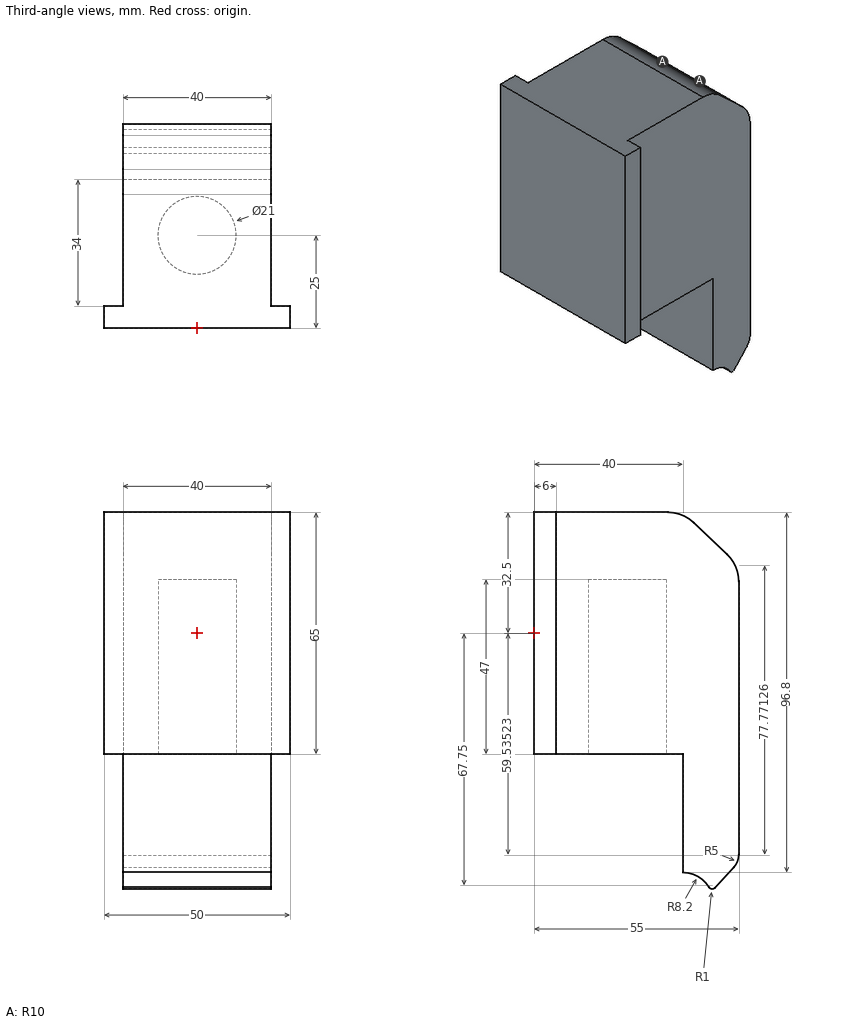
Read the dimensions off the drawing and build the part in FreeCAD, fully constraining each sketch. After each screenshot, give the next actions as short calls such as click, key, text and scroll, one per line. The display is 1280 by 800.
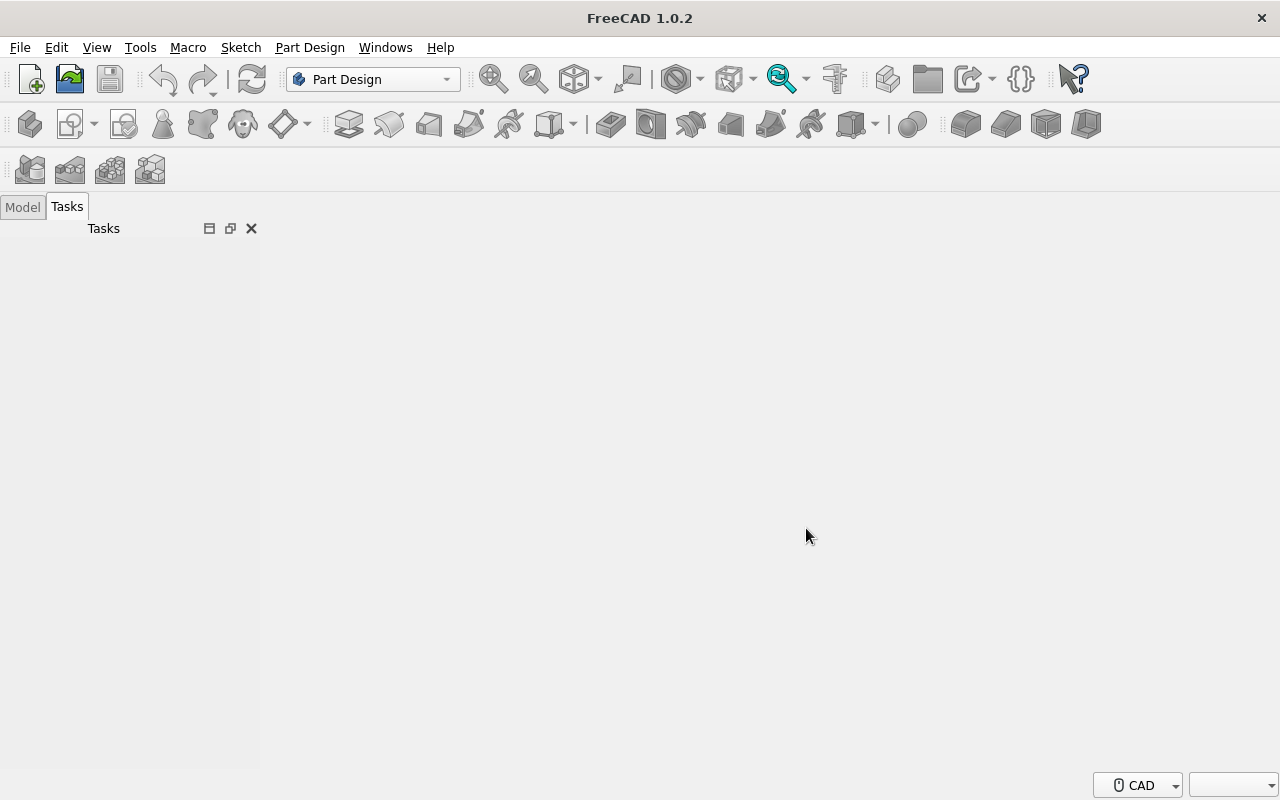
click(30, 80)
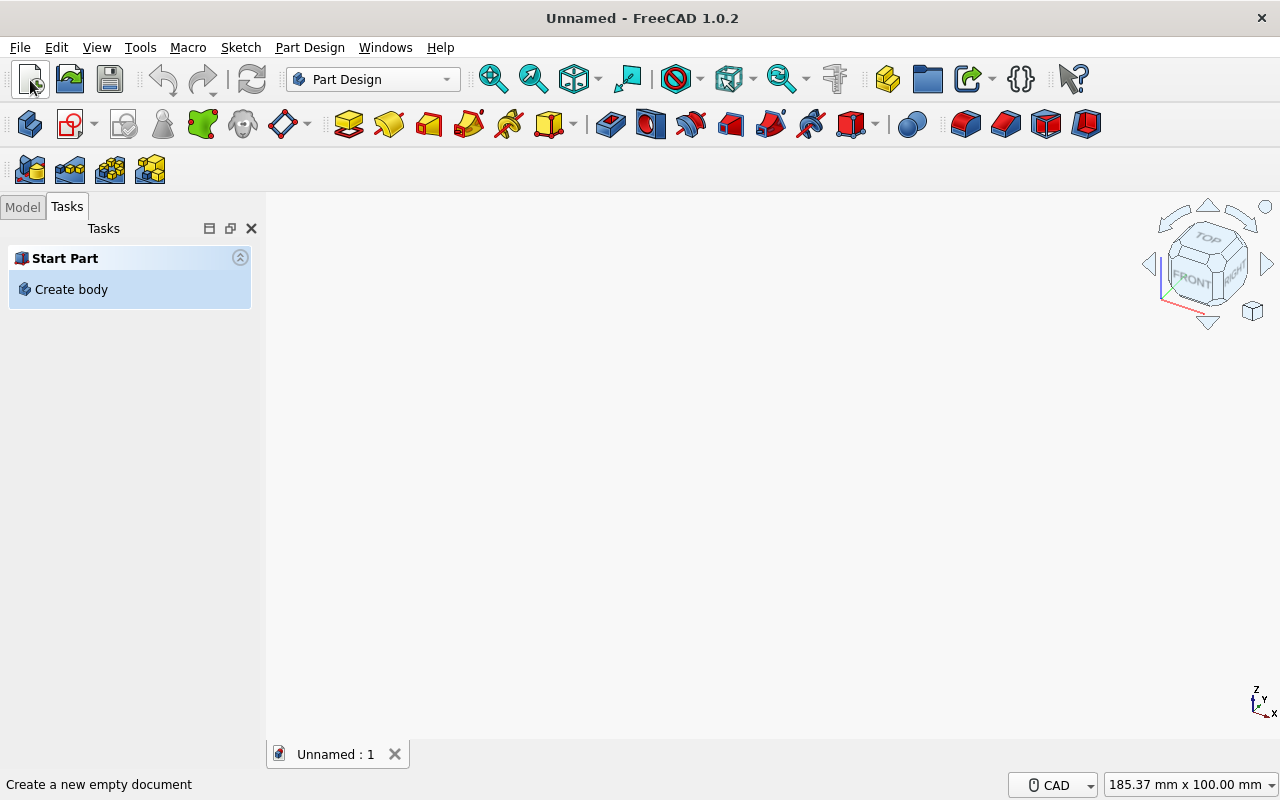
click(70, 124)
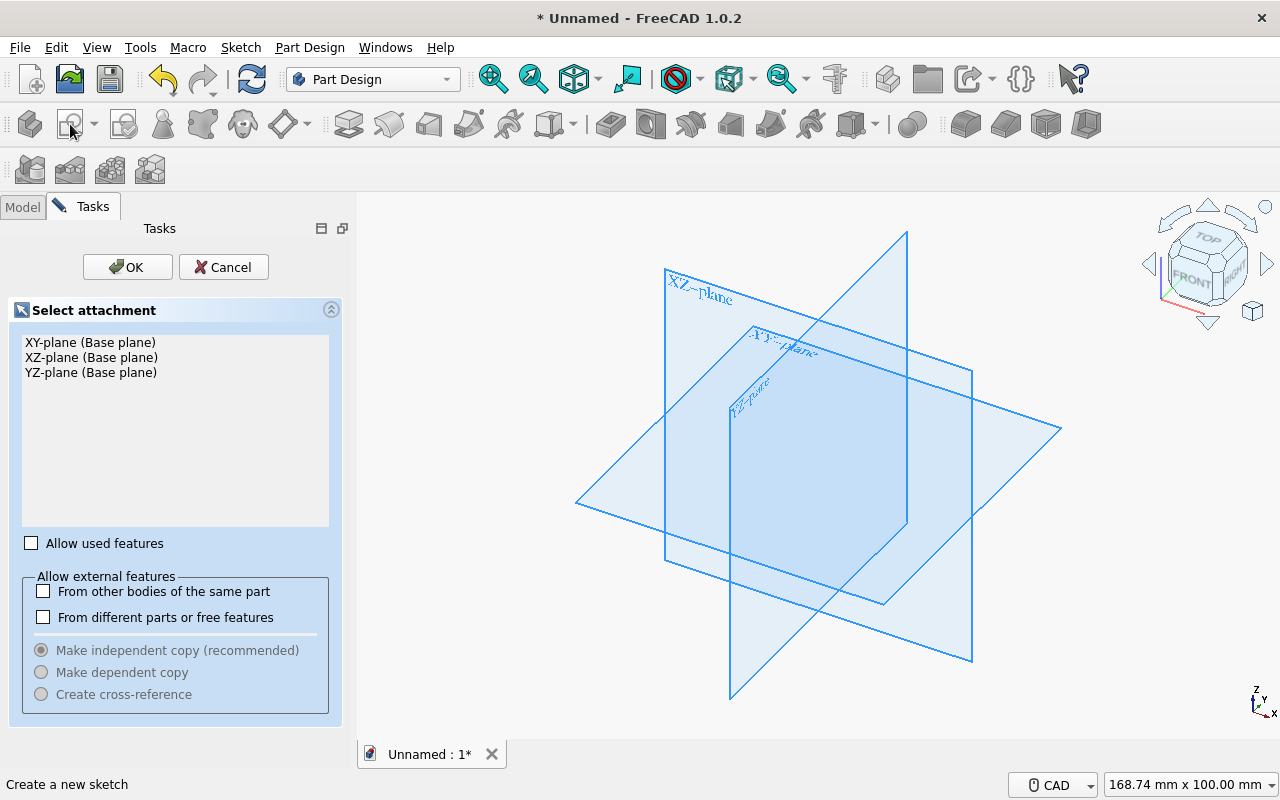
click(82, 358)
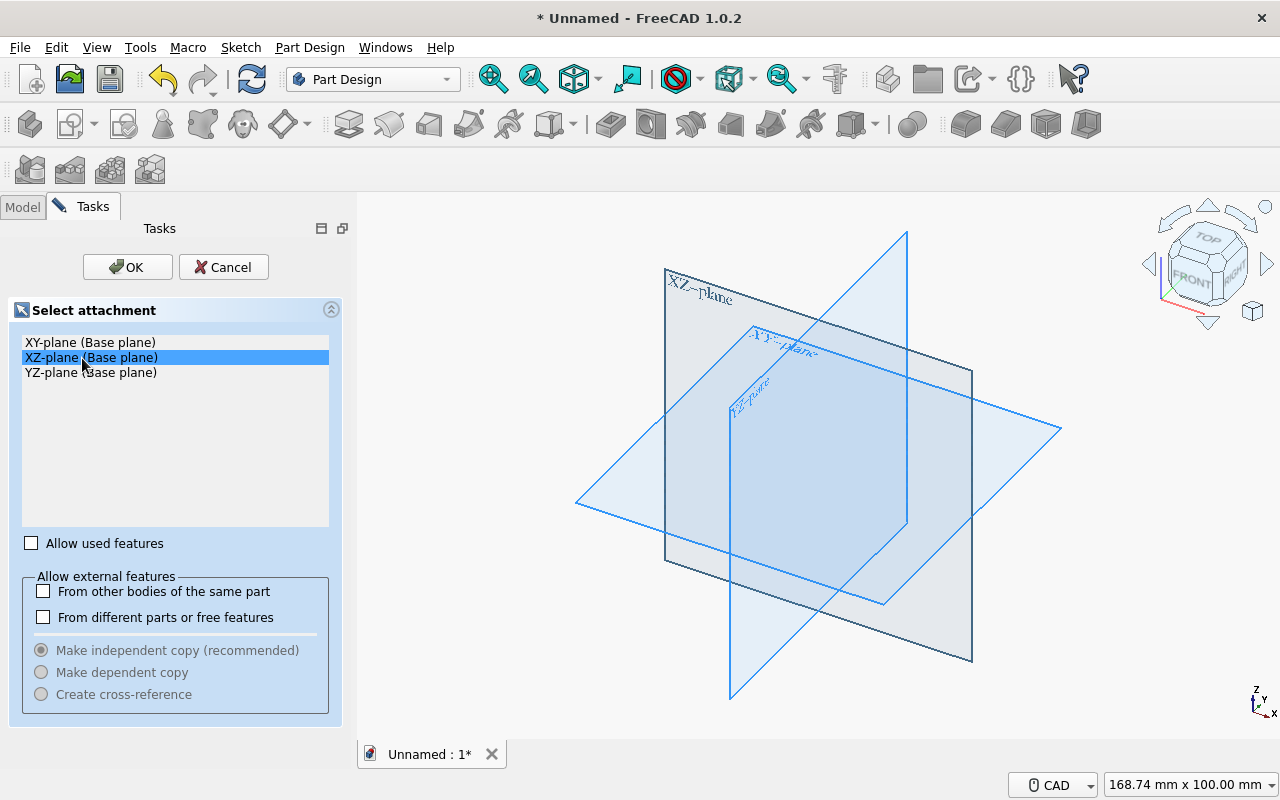
click(128, 267)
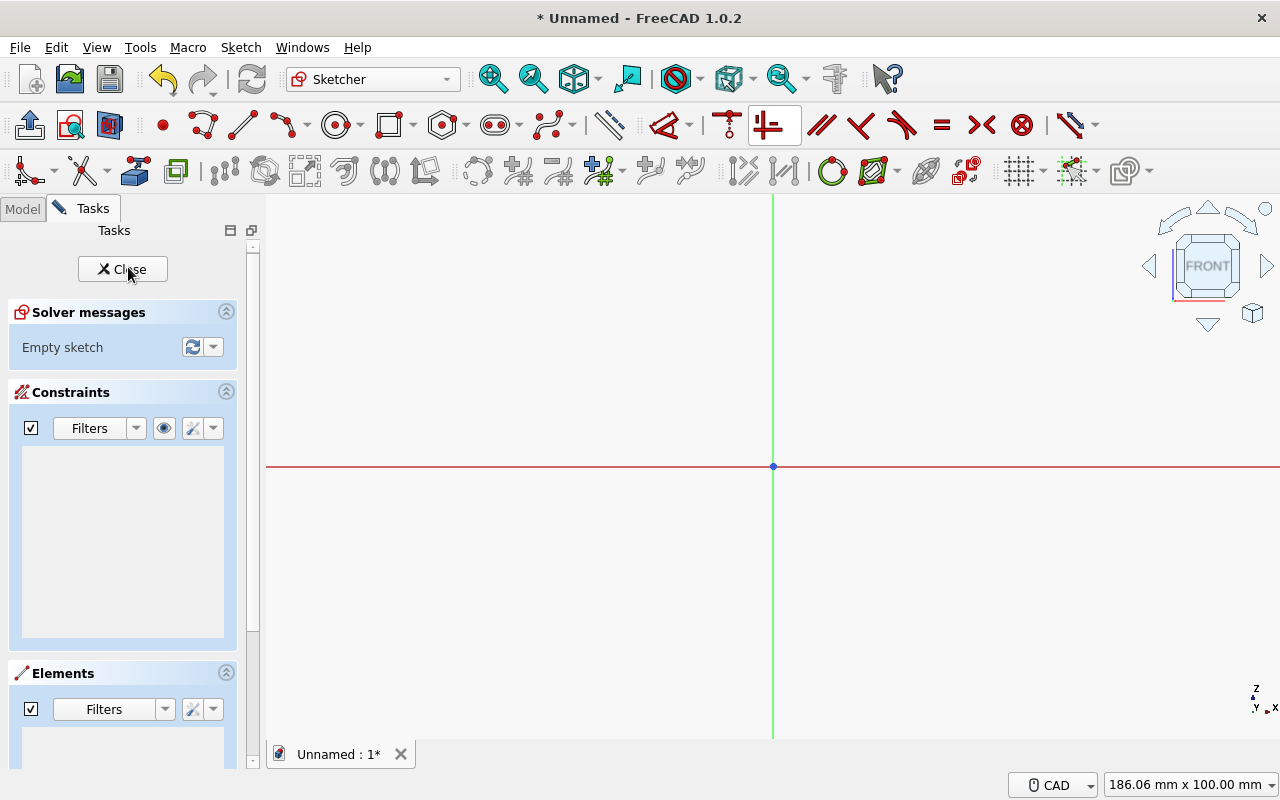
key(g)
key(v)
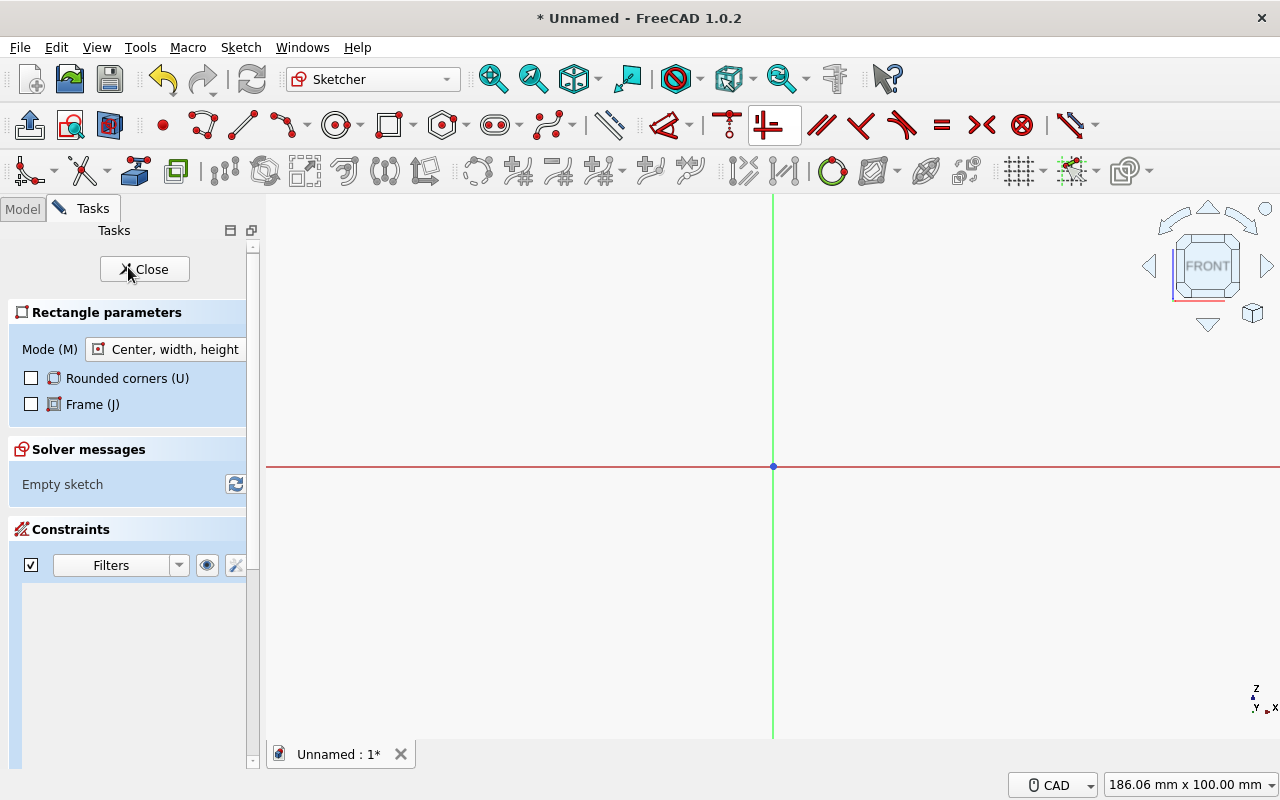
click(773, 466)
move(909, 289)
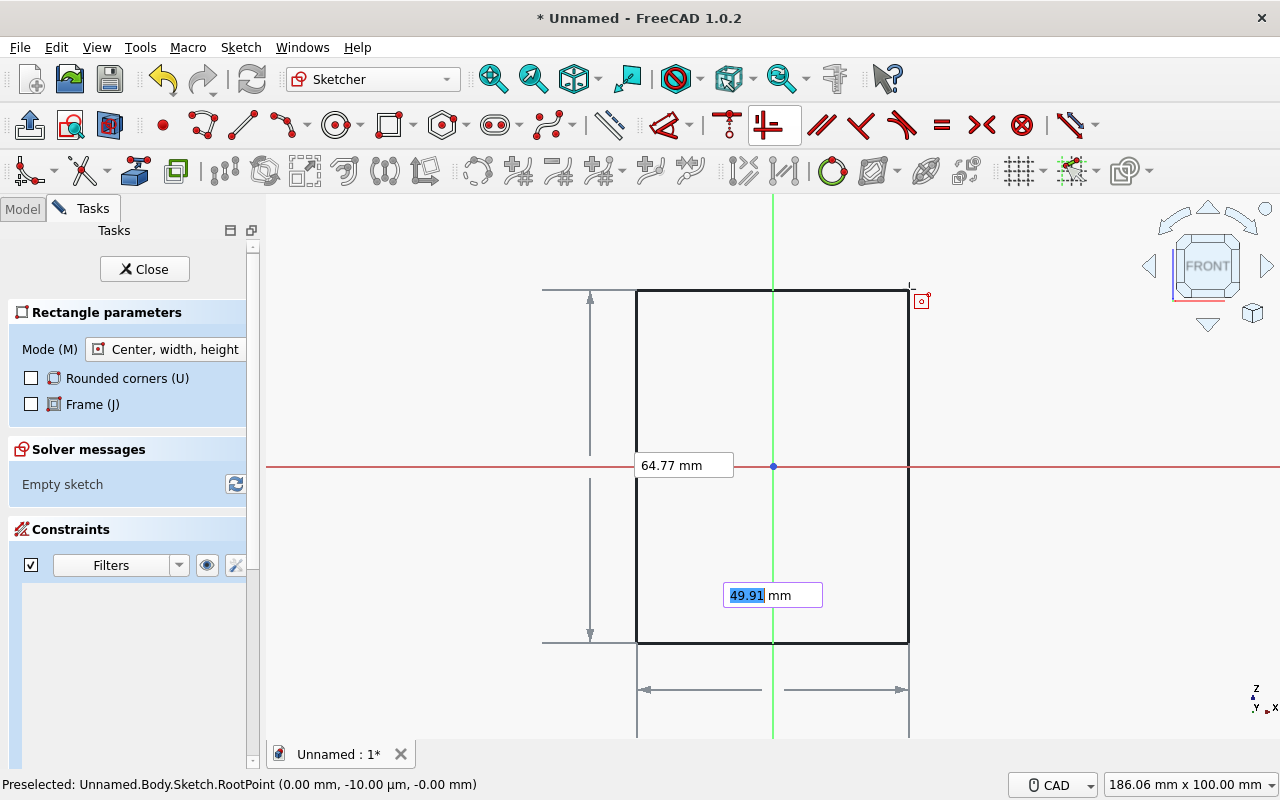
text(50)
key(Tab)
text(65)
key(Return)
key(Escape)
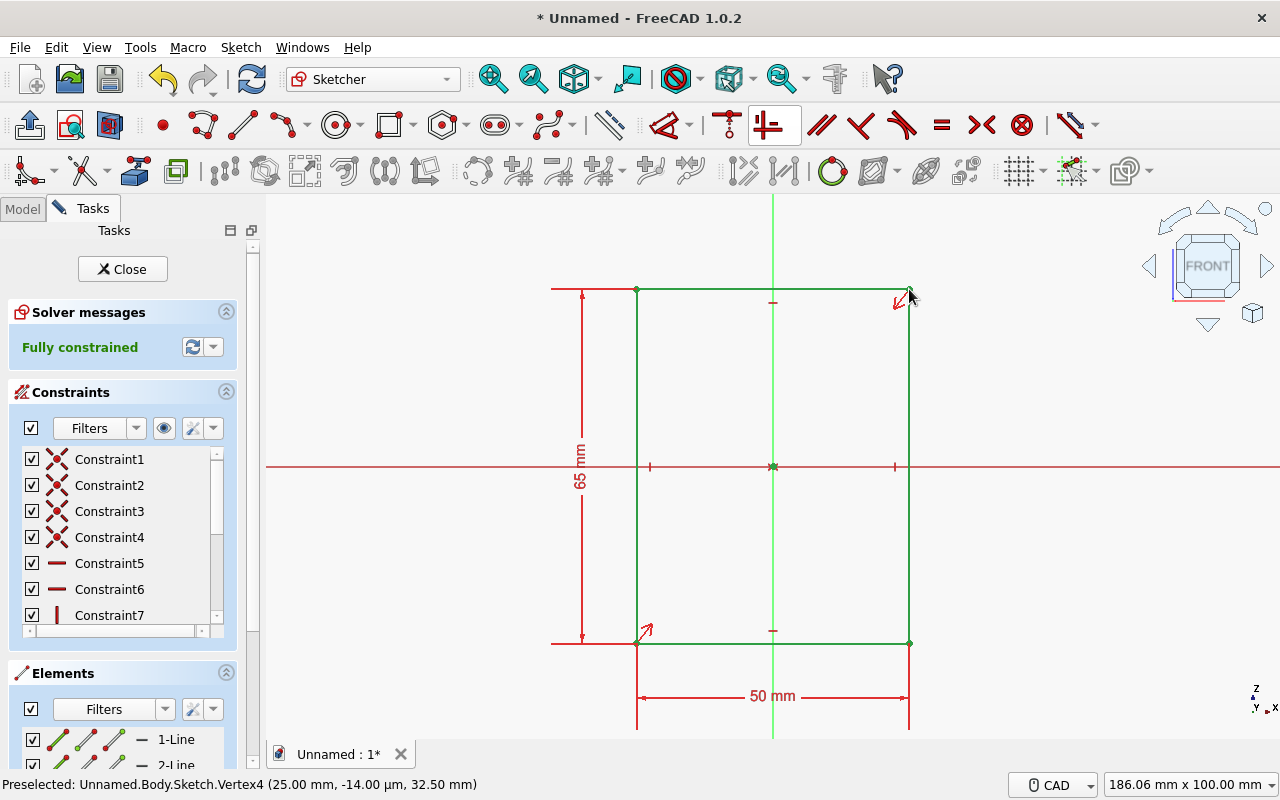
click(123, 269)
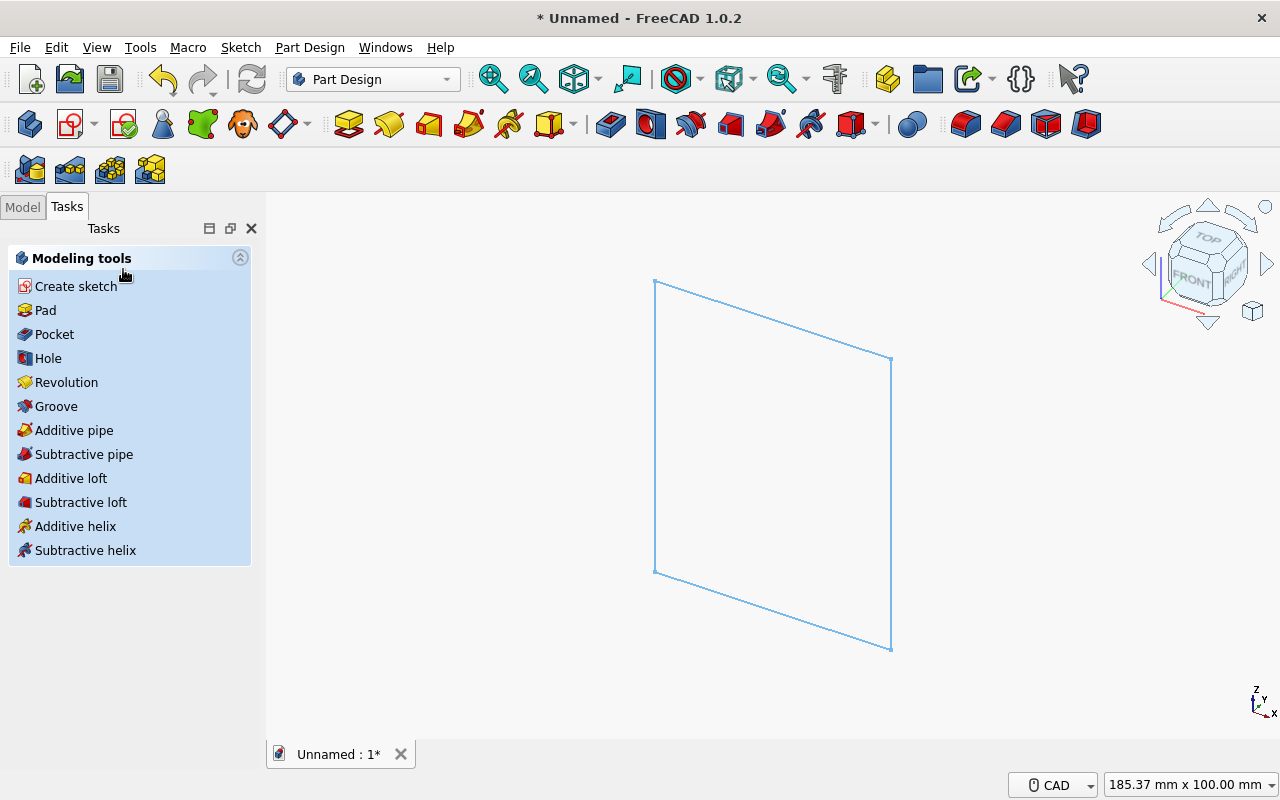
click(350, 124)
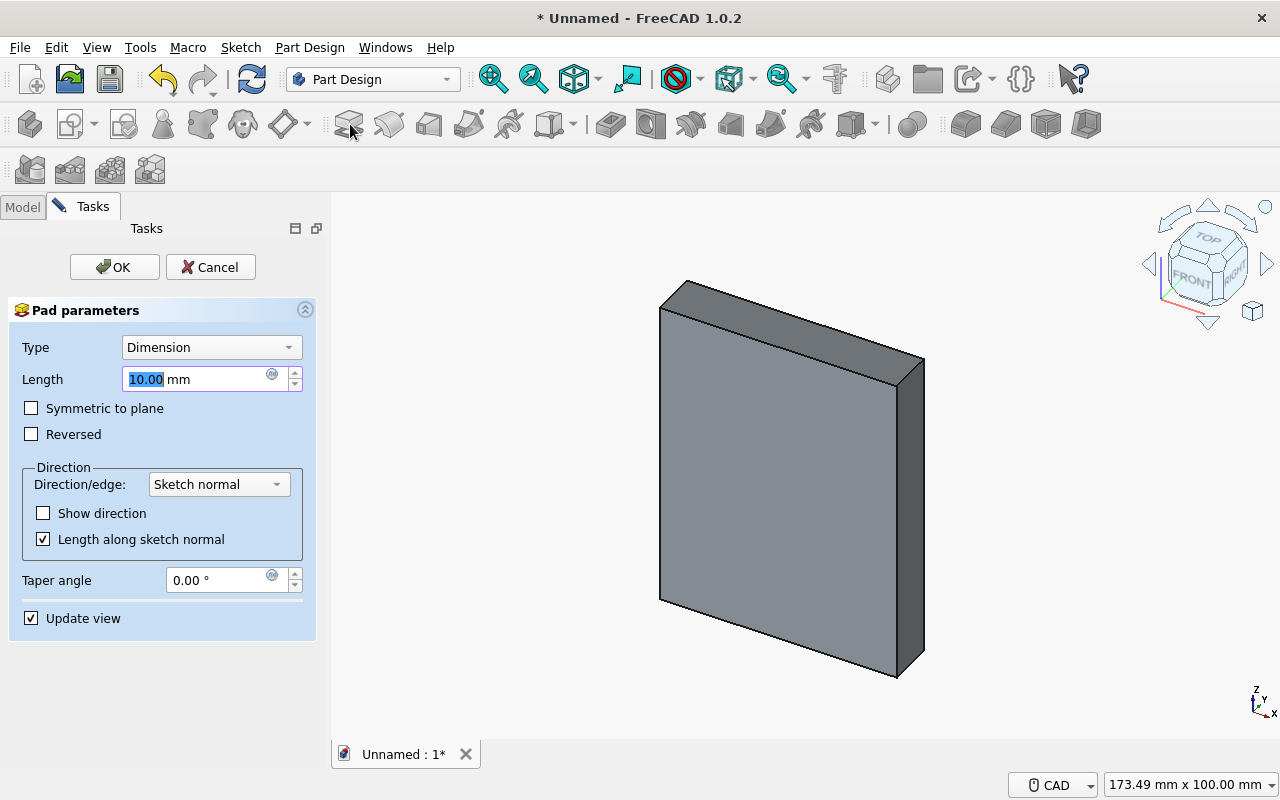
text(6)
key(Tab)